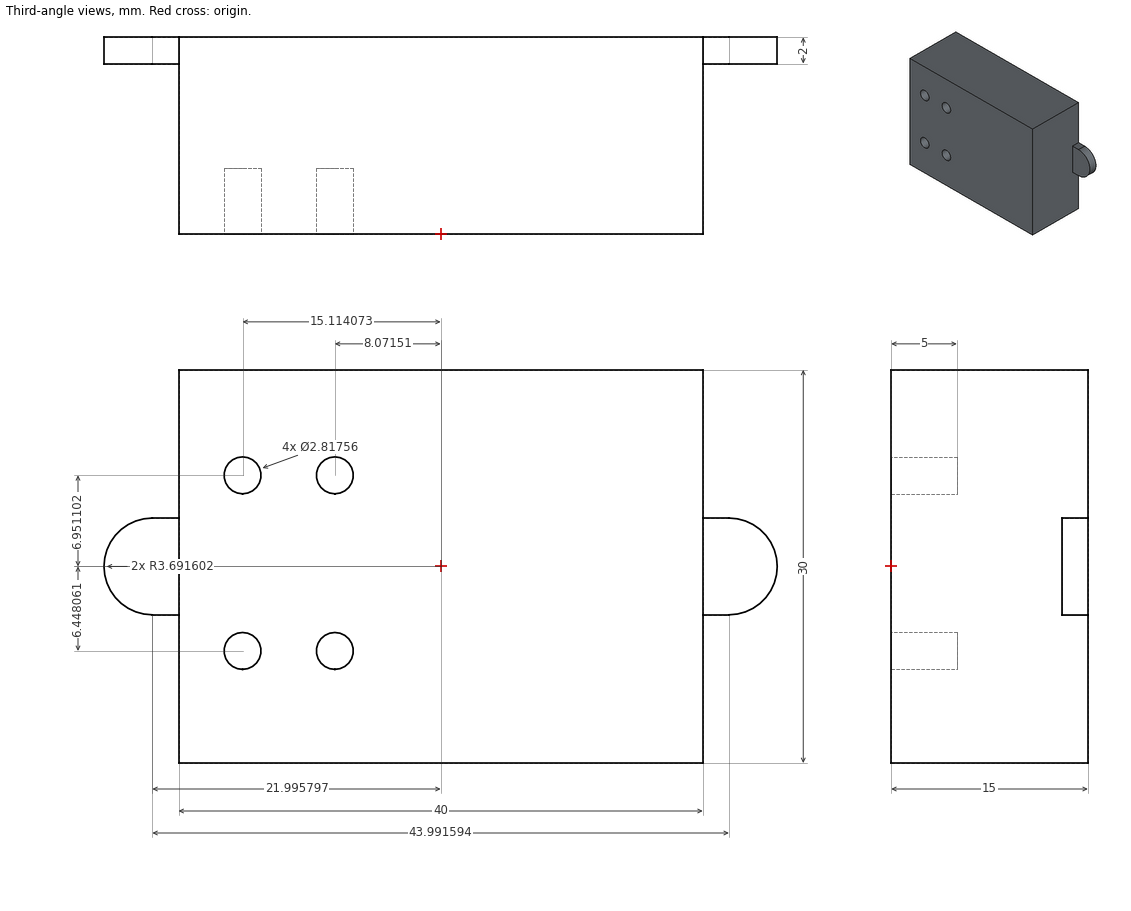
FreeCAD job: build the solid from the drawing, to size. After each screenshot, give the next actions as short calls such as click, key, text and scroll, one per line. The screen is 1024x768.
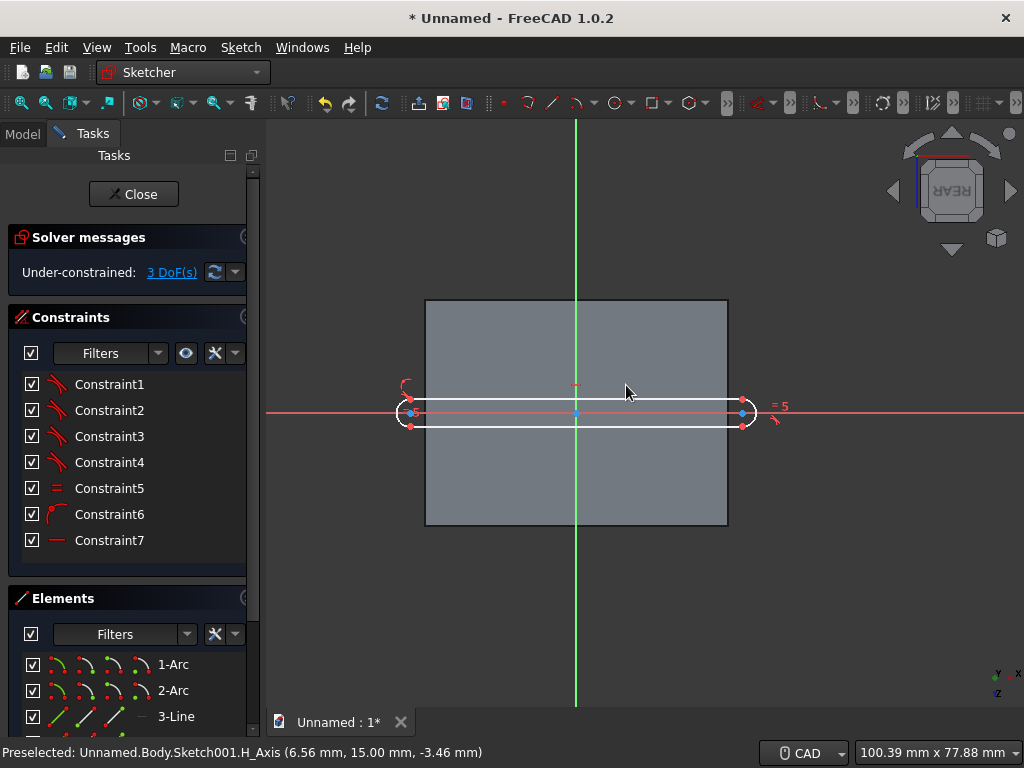
click(758, 104)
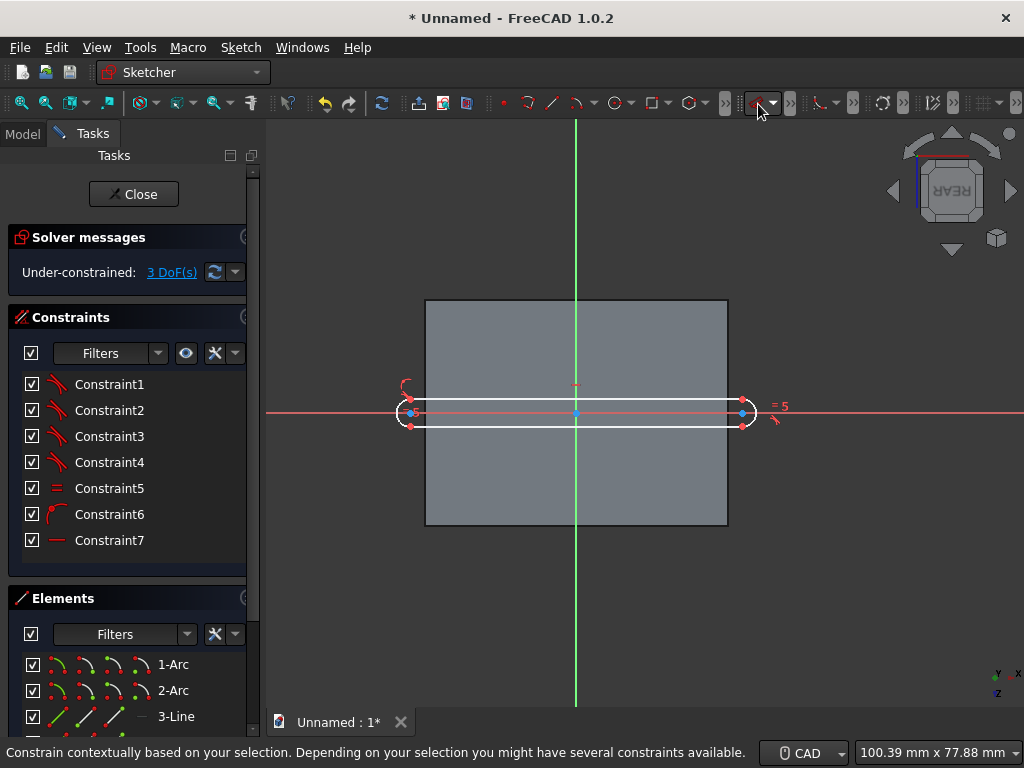
scroll(397, 413, up, 2)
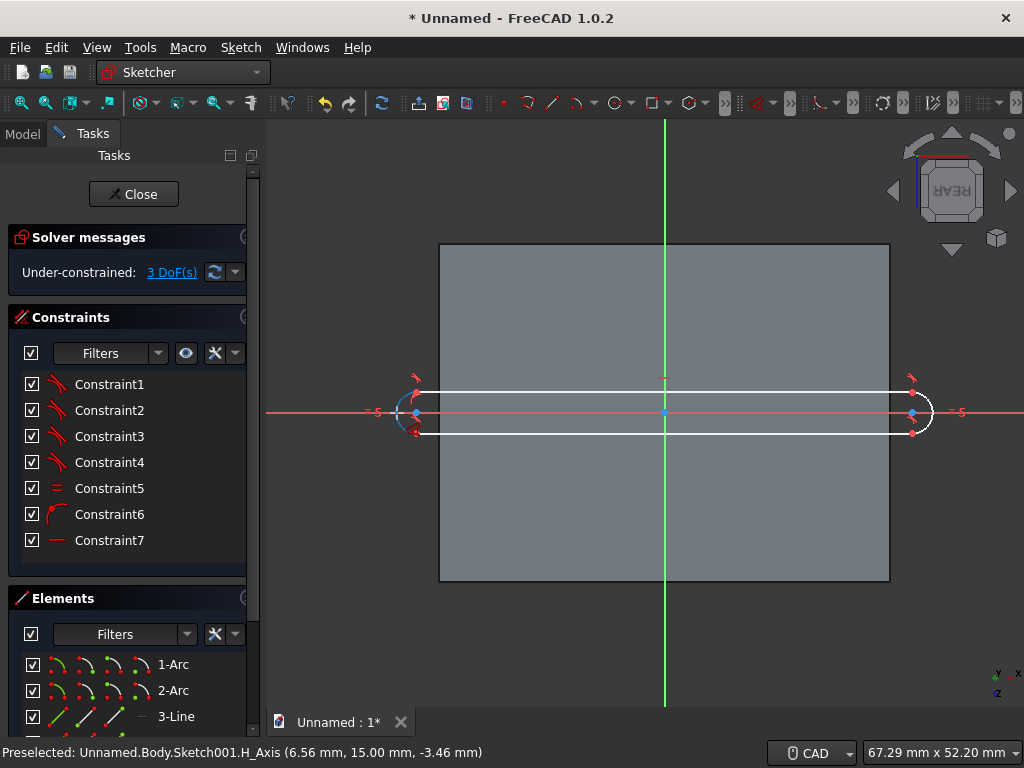
click(396, 413)
click(370, 388)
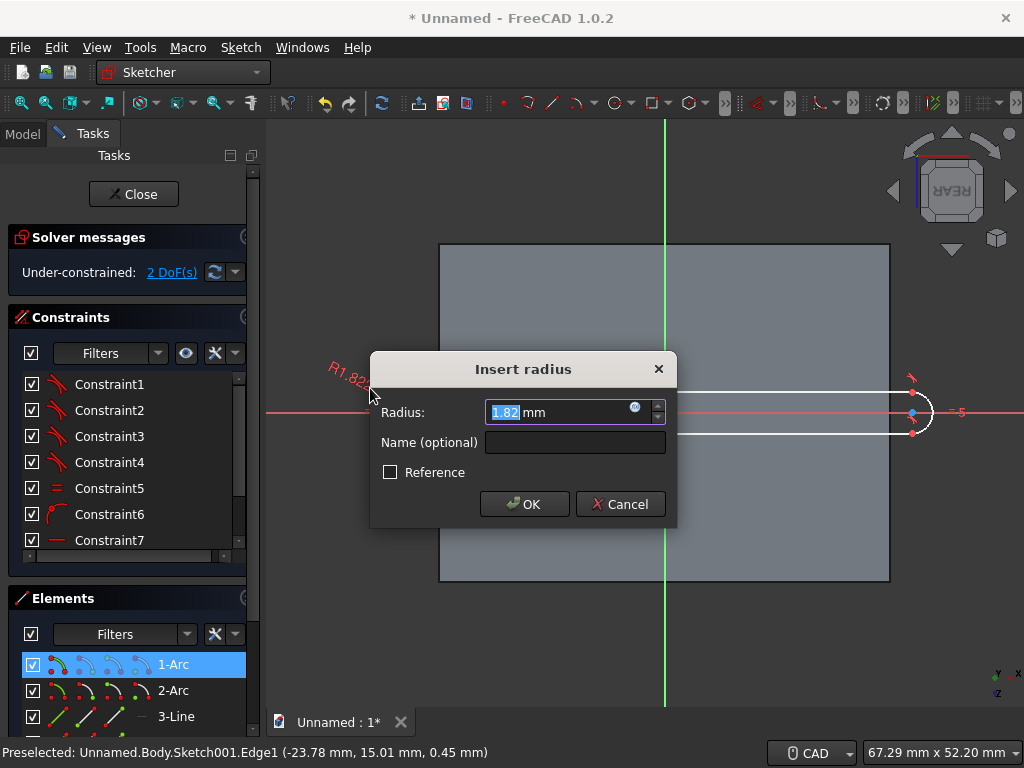
text(3.691602)
key(Return)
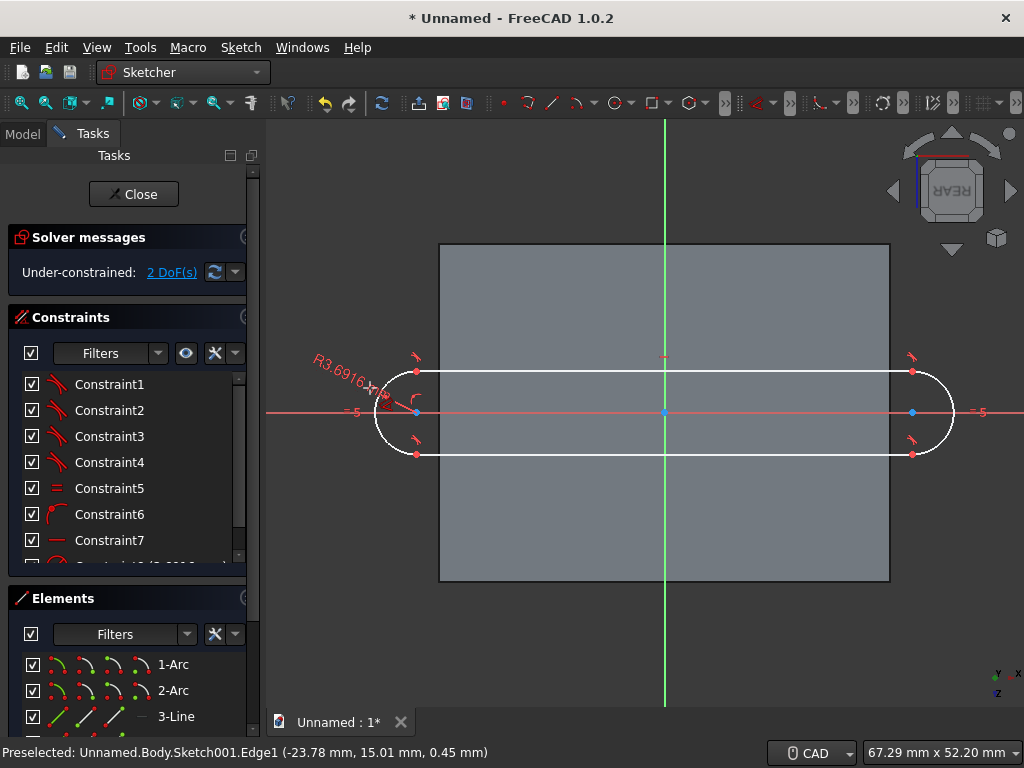
click(565, 371)
click(638, 337)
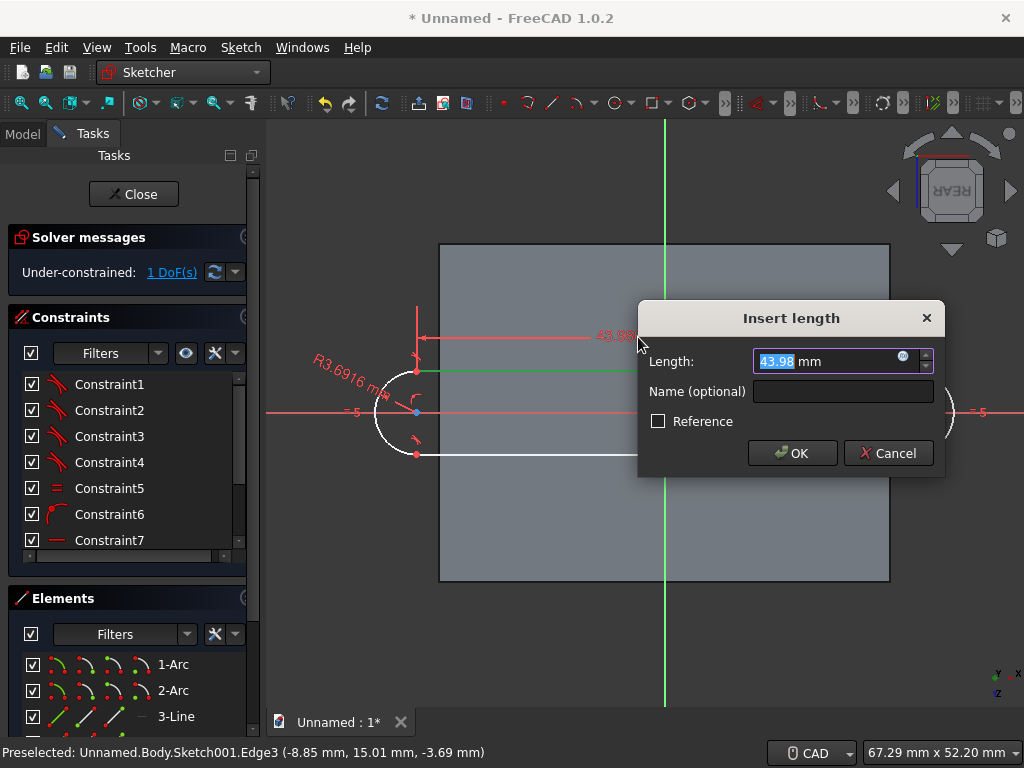
text(43.991594)
key(Return)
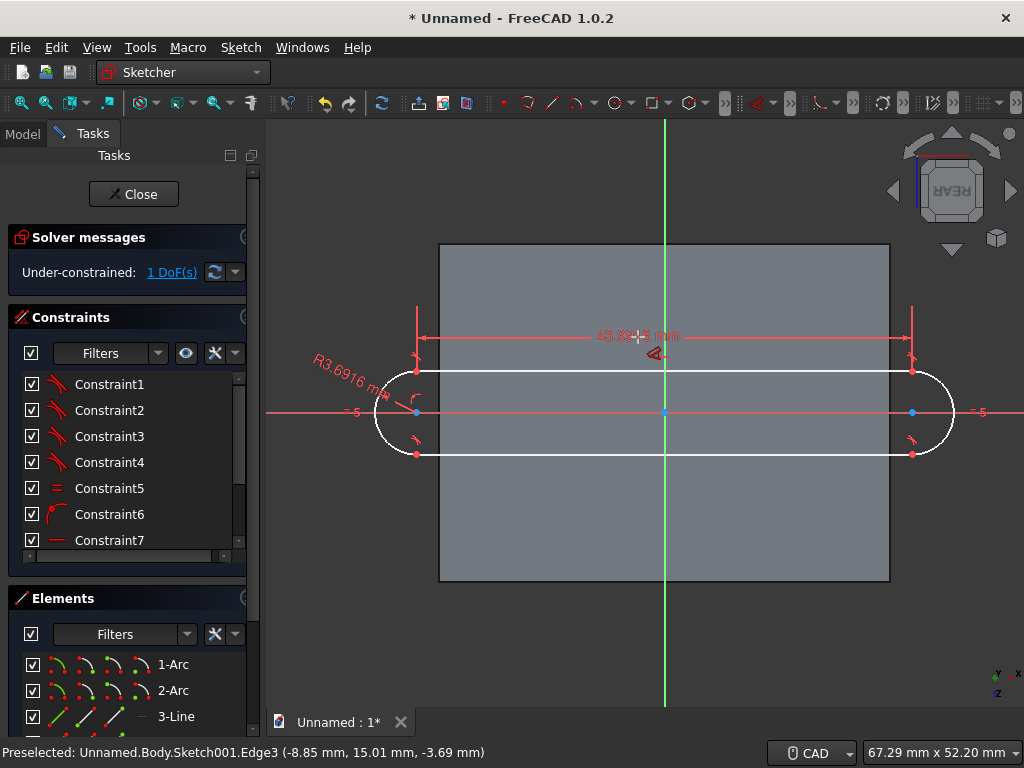
click(417, 371)
click(541, 337)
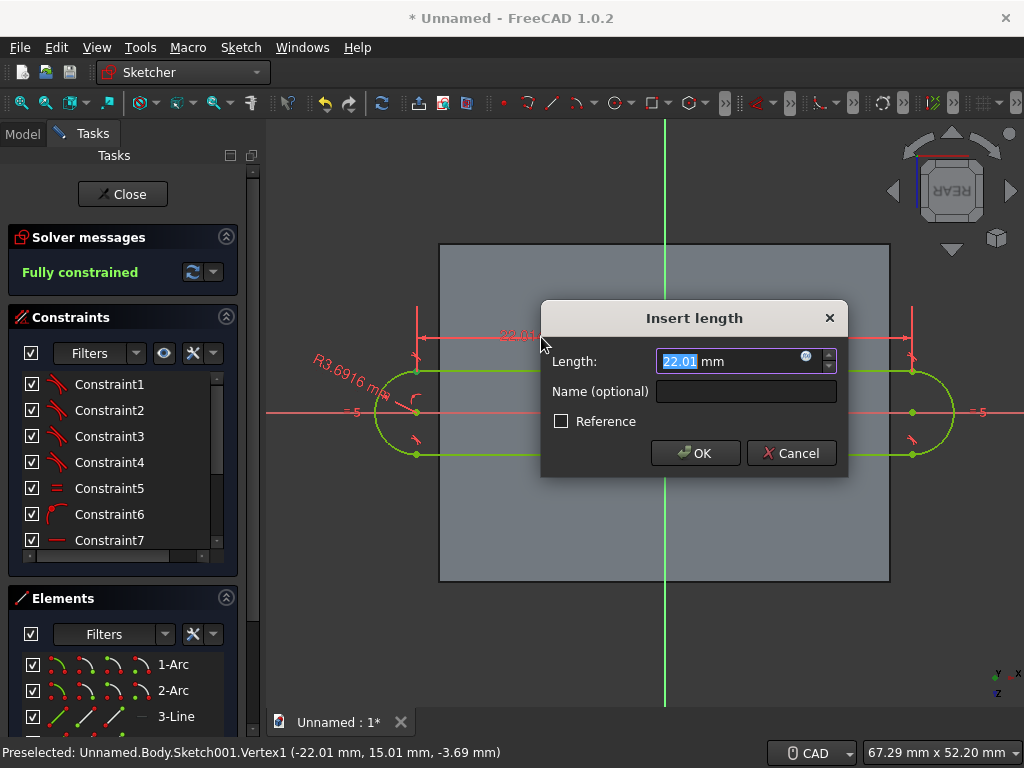
text(21.995797)
key(Return)
key(Escape)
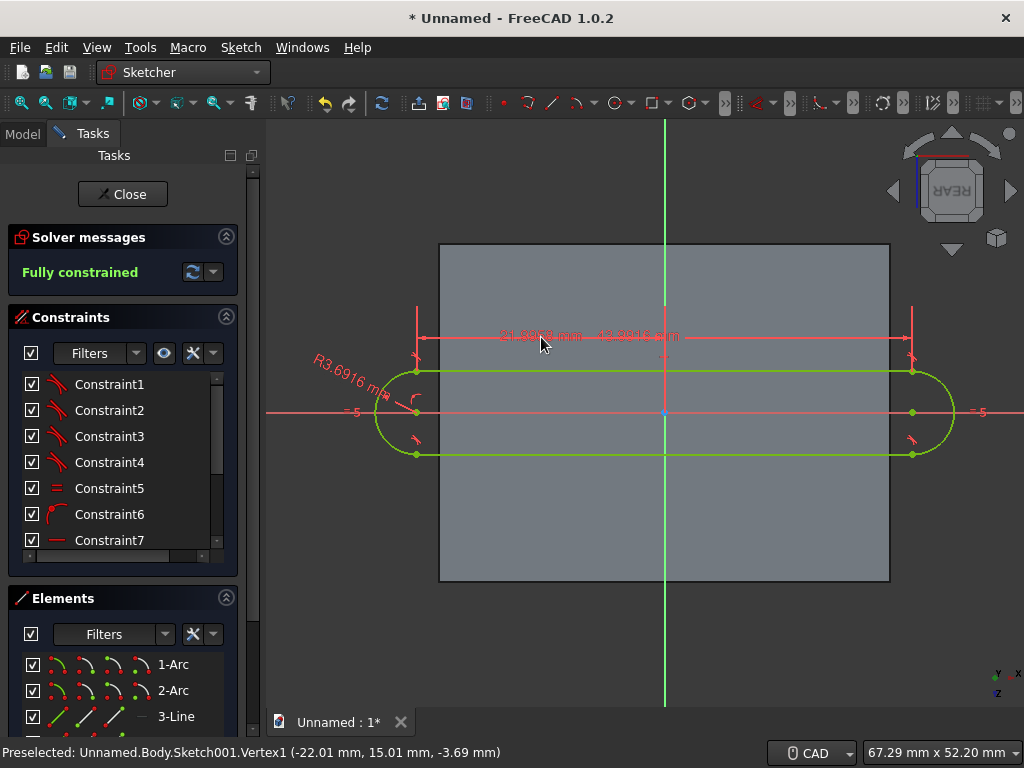
click(123, 194)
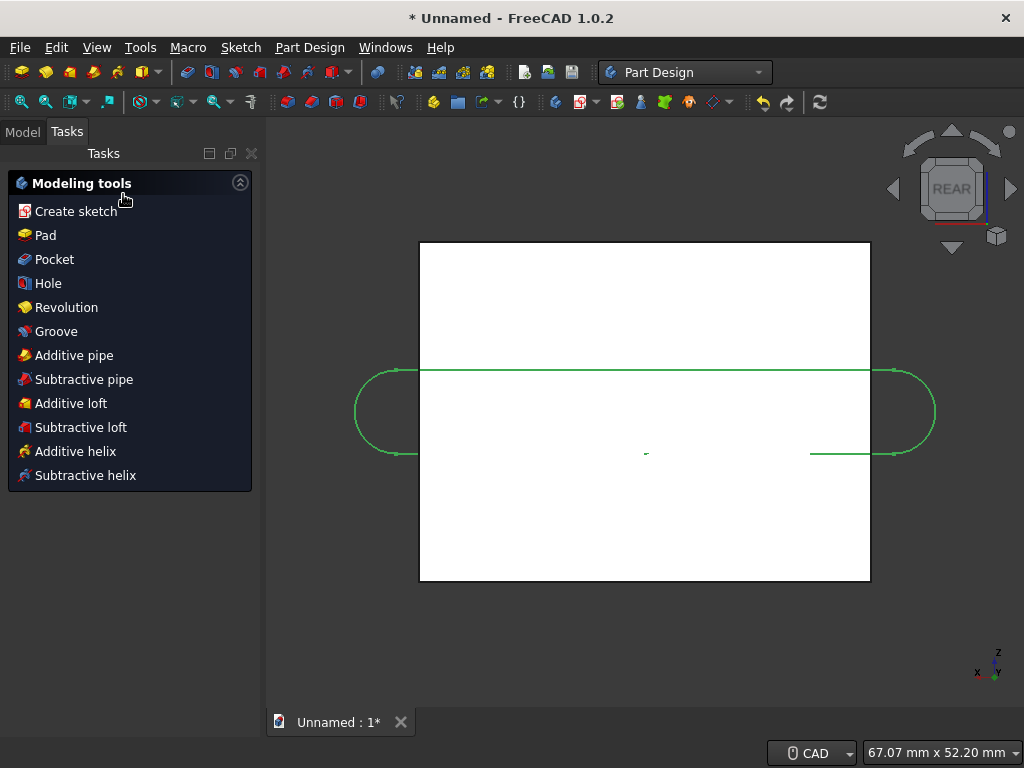
click(22, 72)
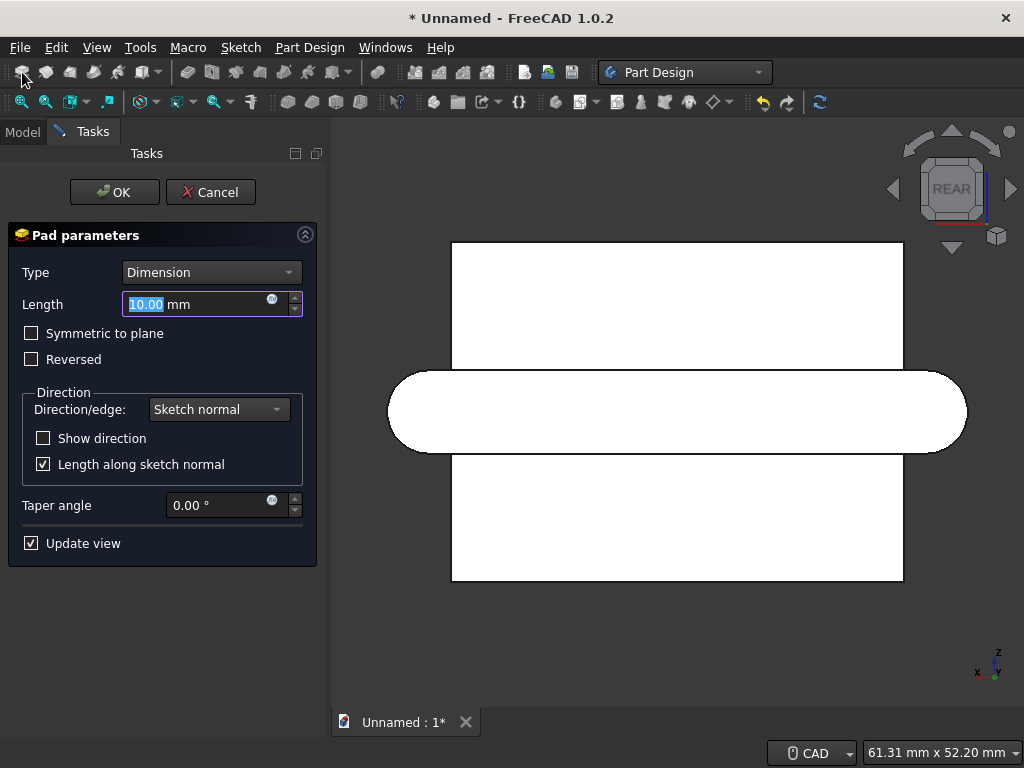
text(2)
key(Tab)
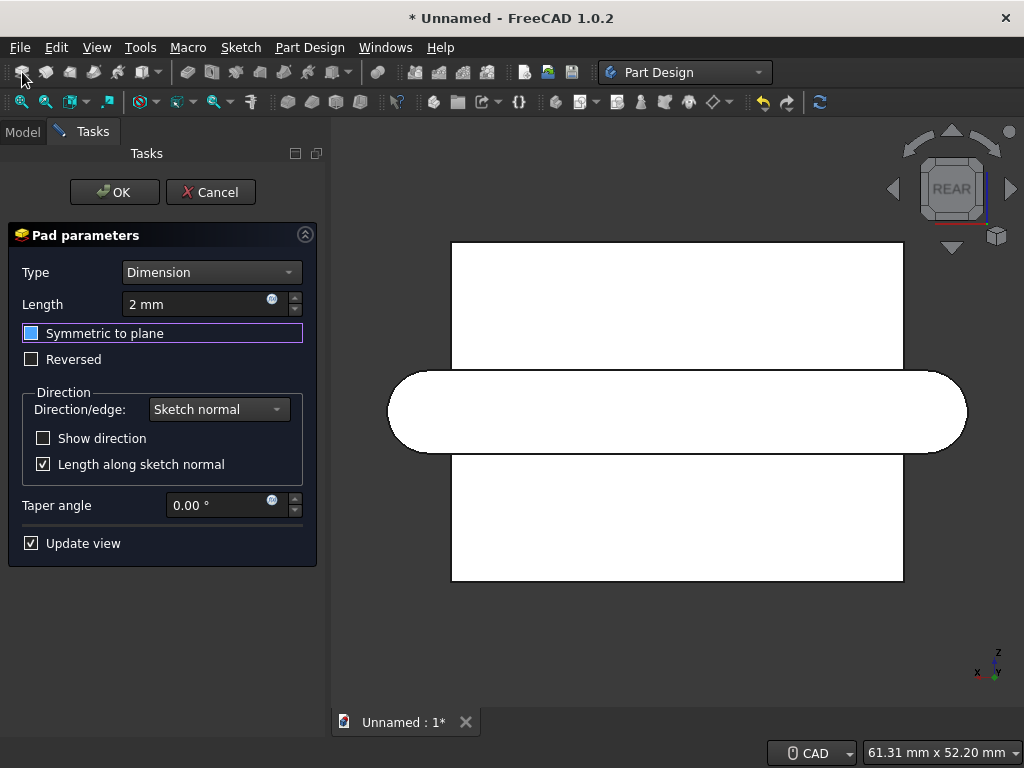
click(30, 359)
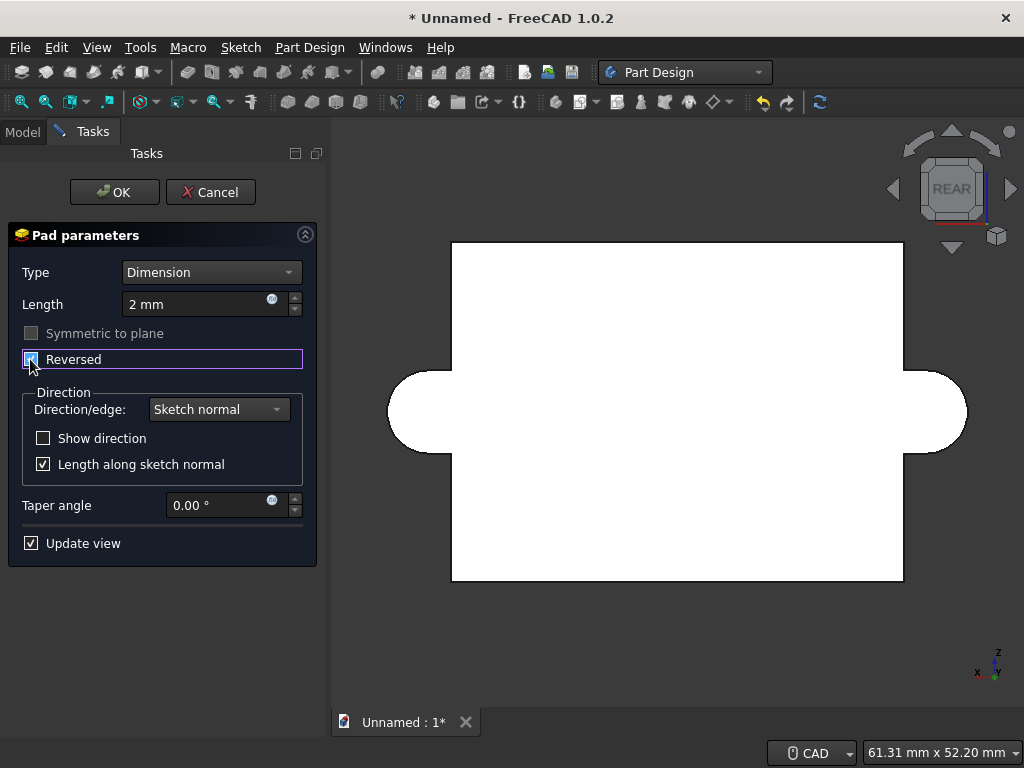
click(115, 192)